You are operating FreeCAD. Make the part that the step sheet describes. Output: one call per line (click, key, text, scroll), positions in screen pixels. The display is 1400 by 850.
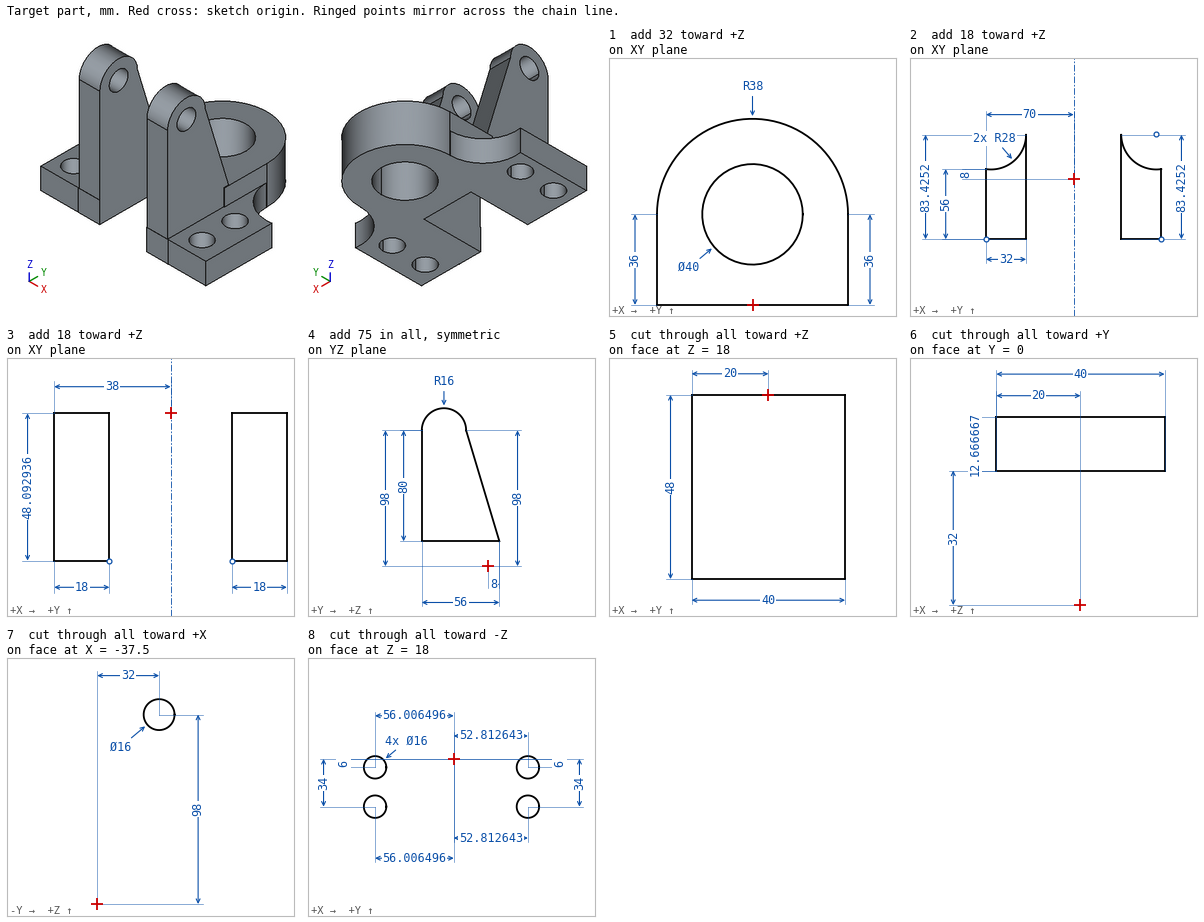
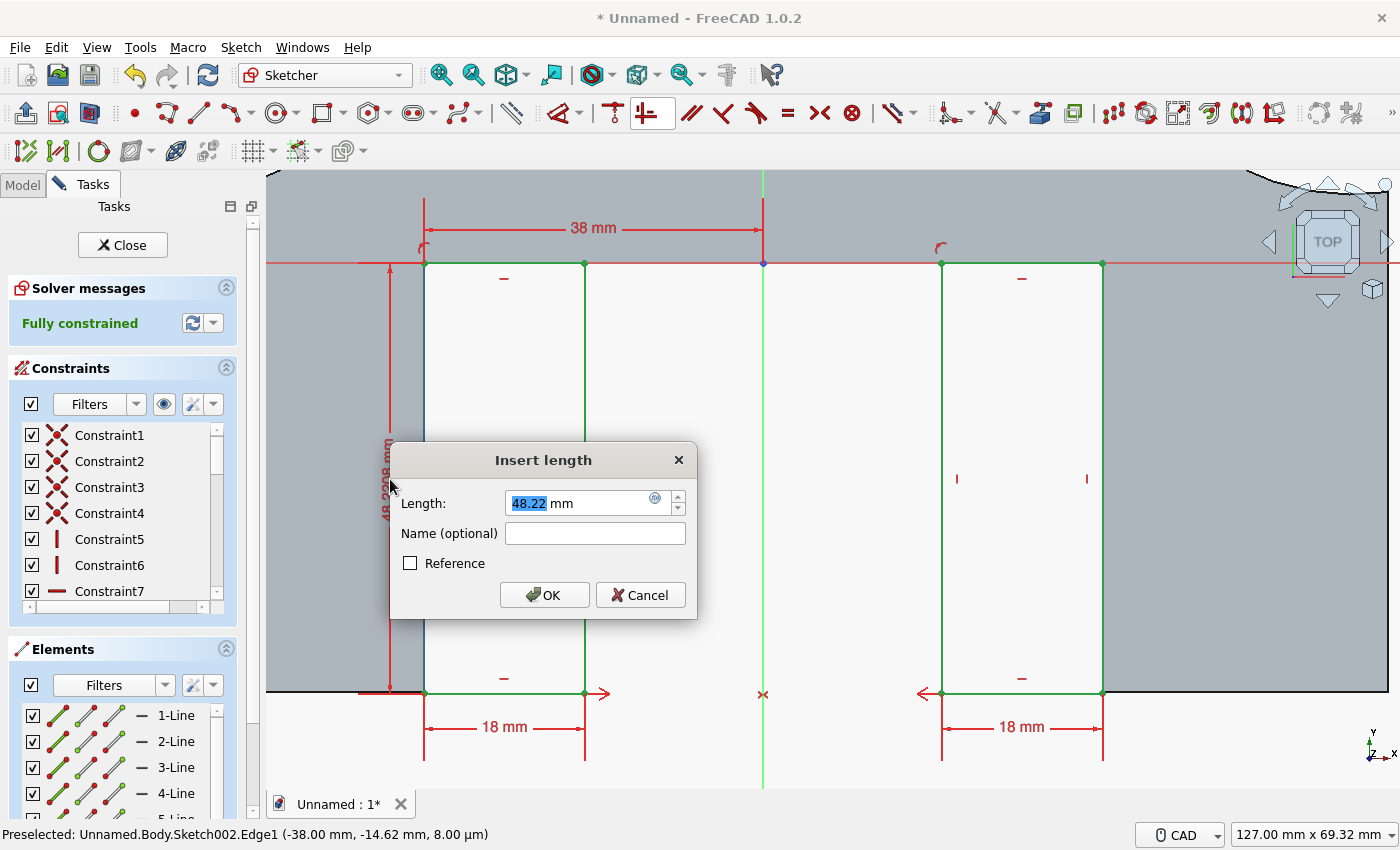
text(48.092936)
key(Return)
key(Escape)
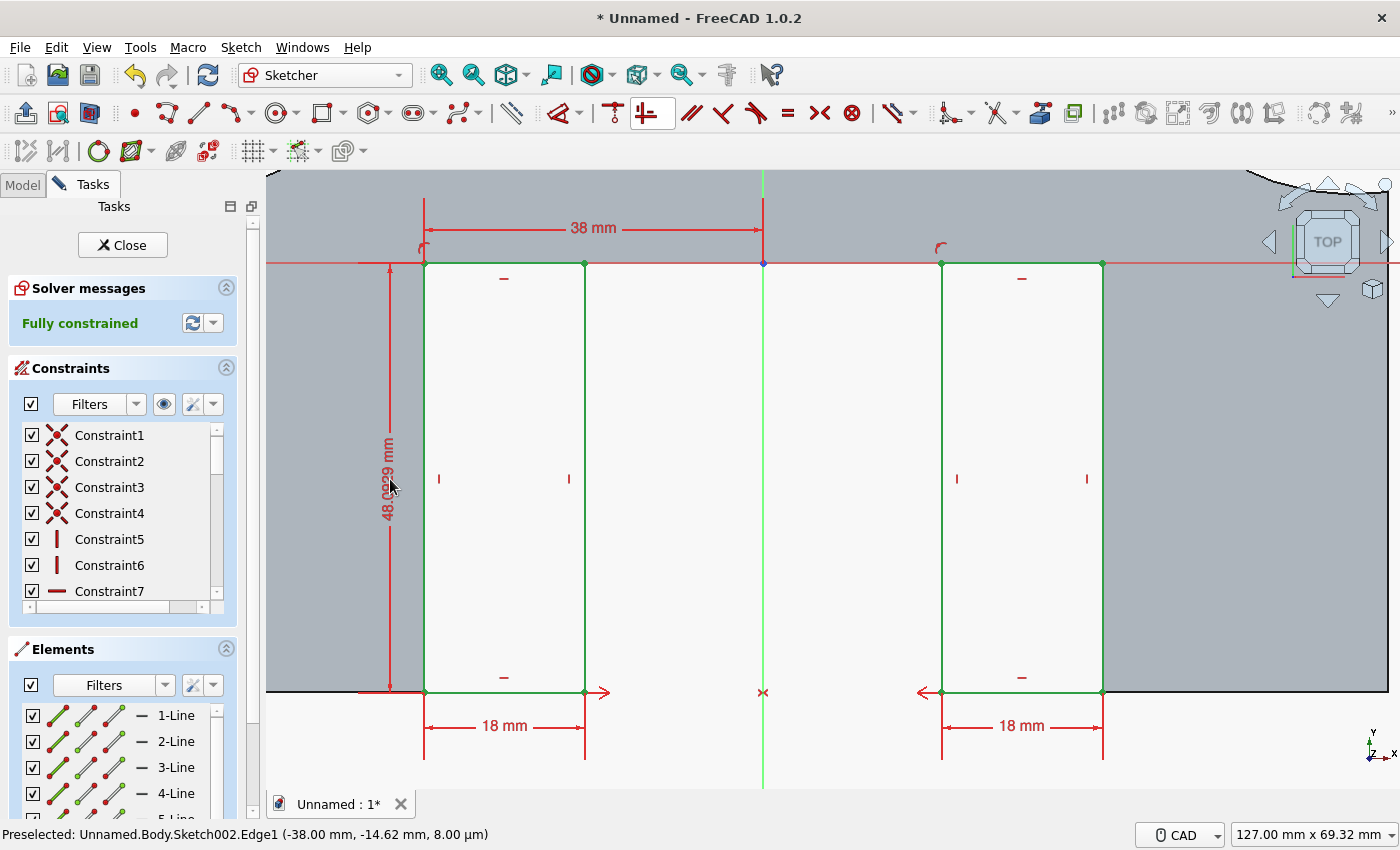
click(123, 245)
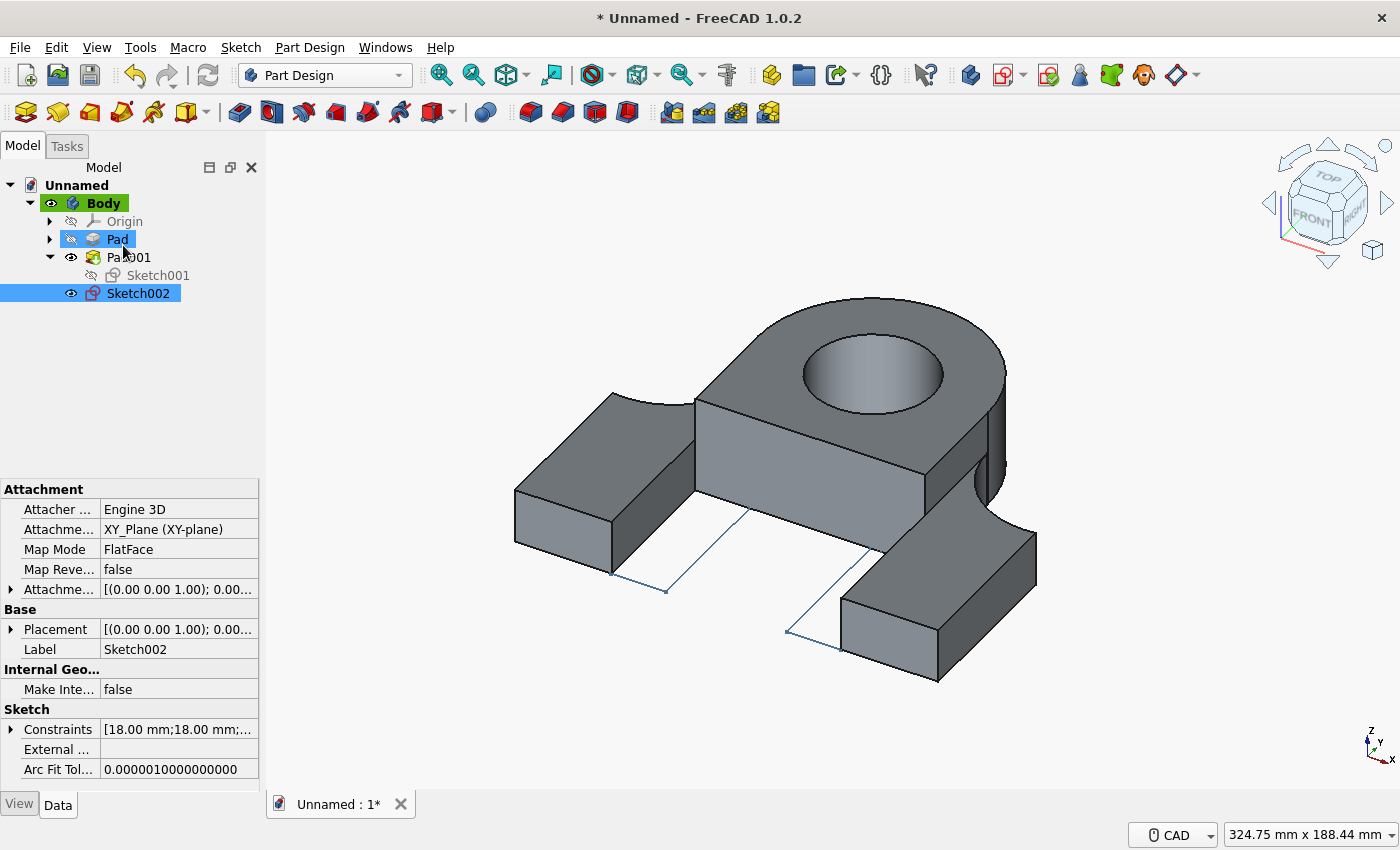
click(26, 112)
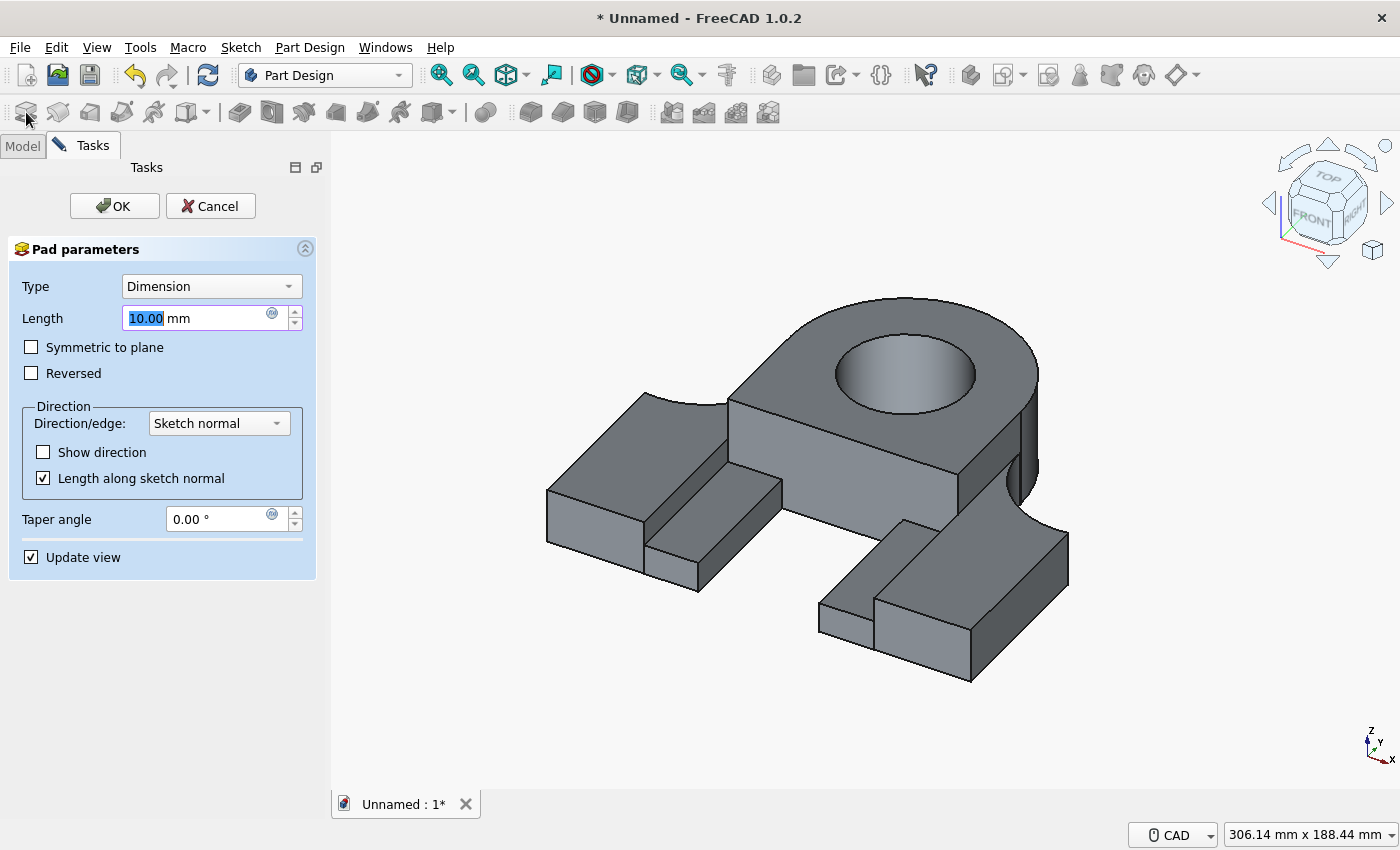
text(18)
key(Tab)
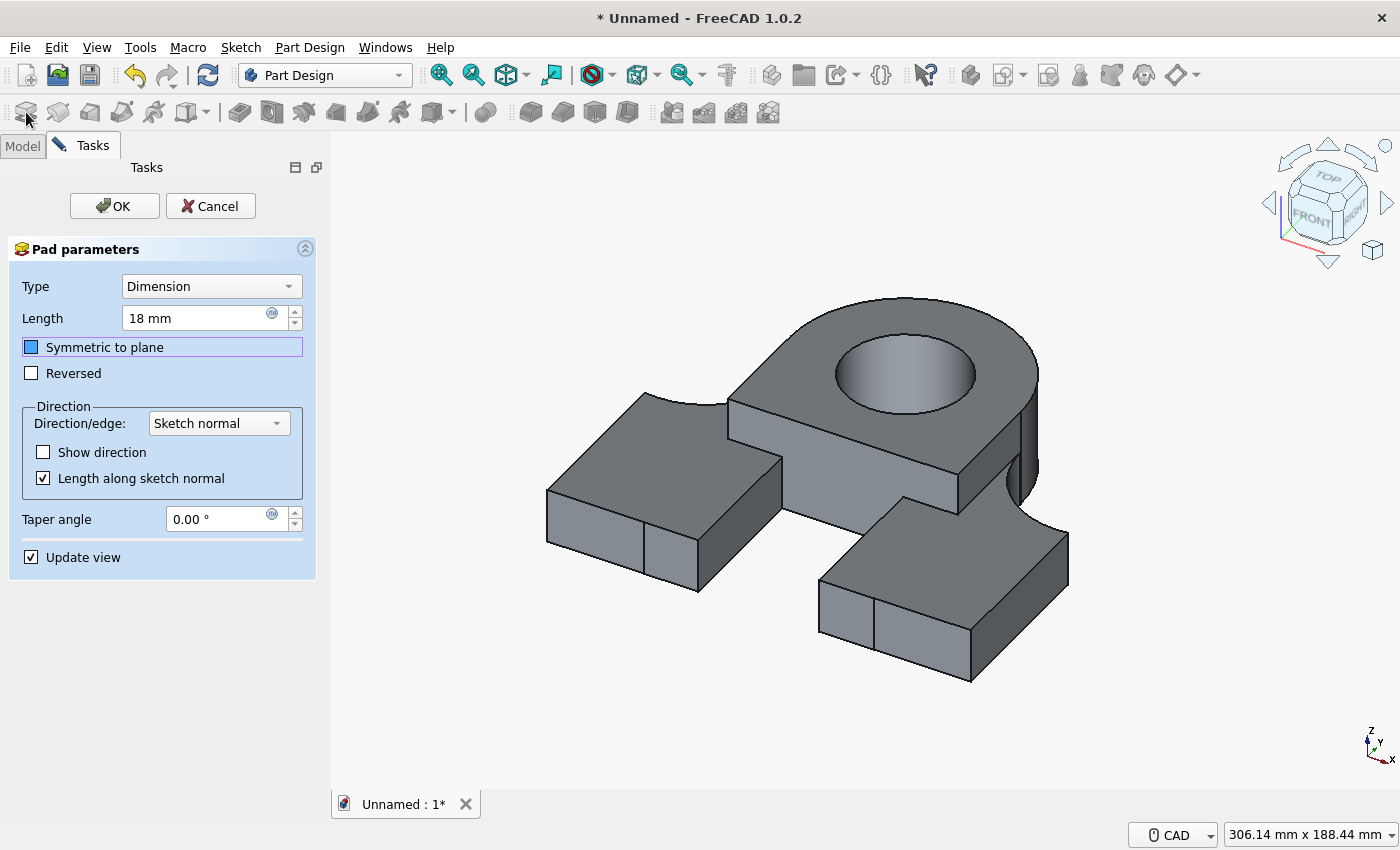
click(115, 206)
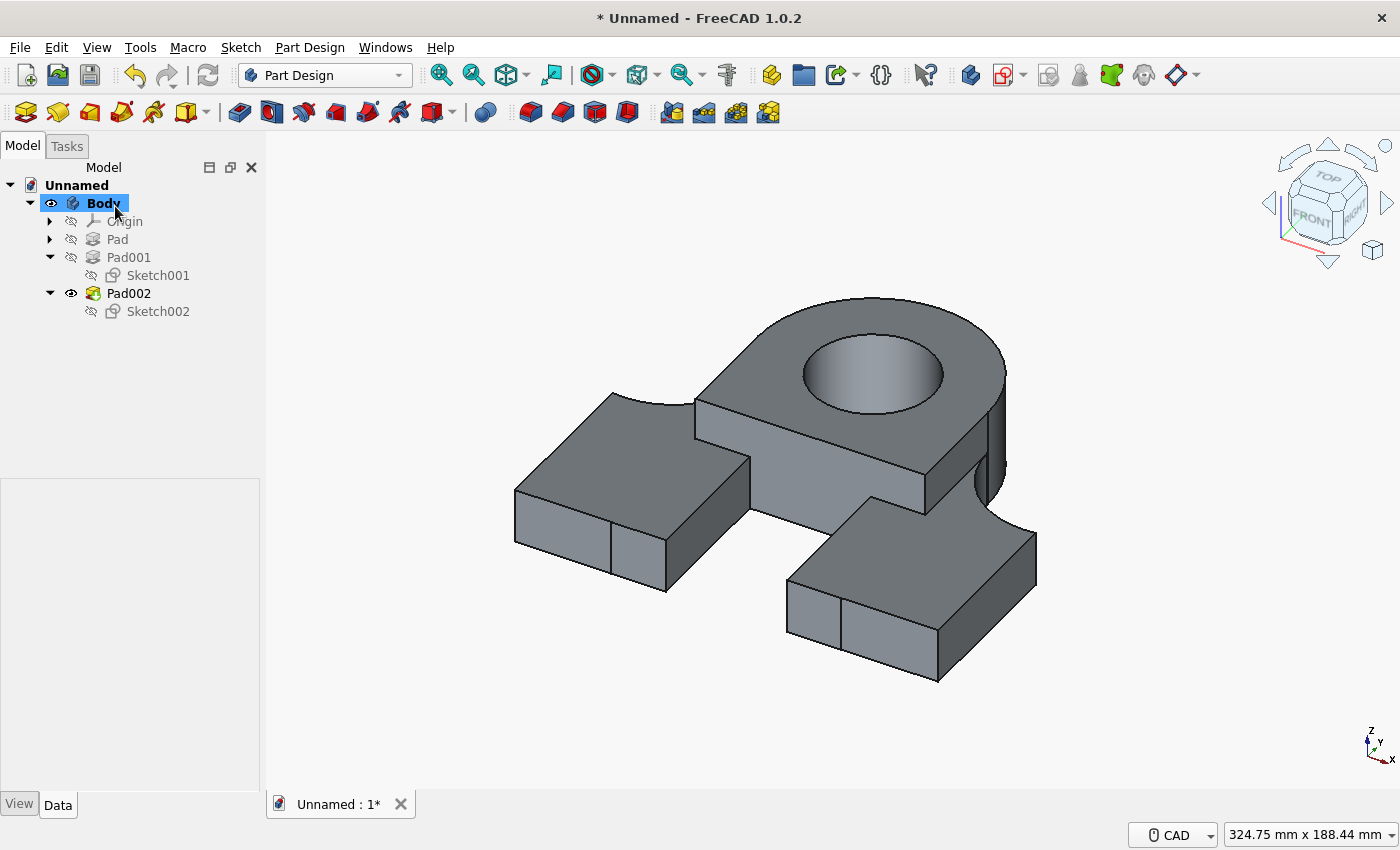
click(1004, 76)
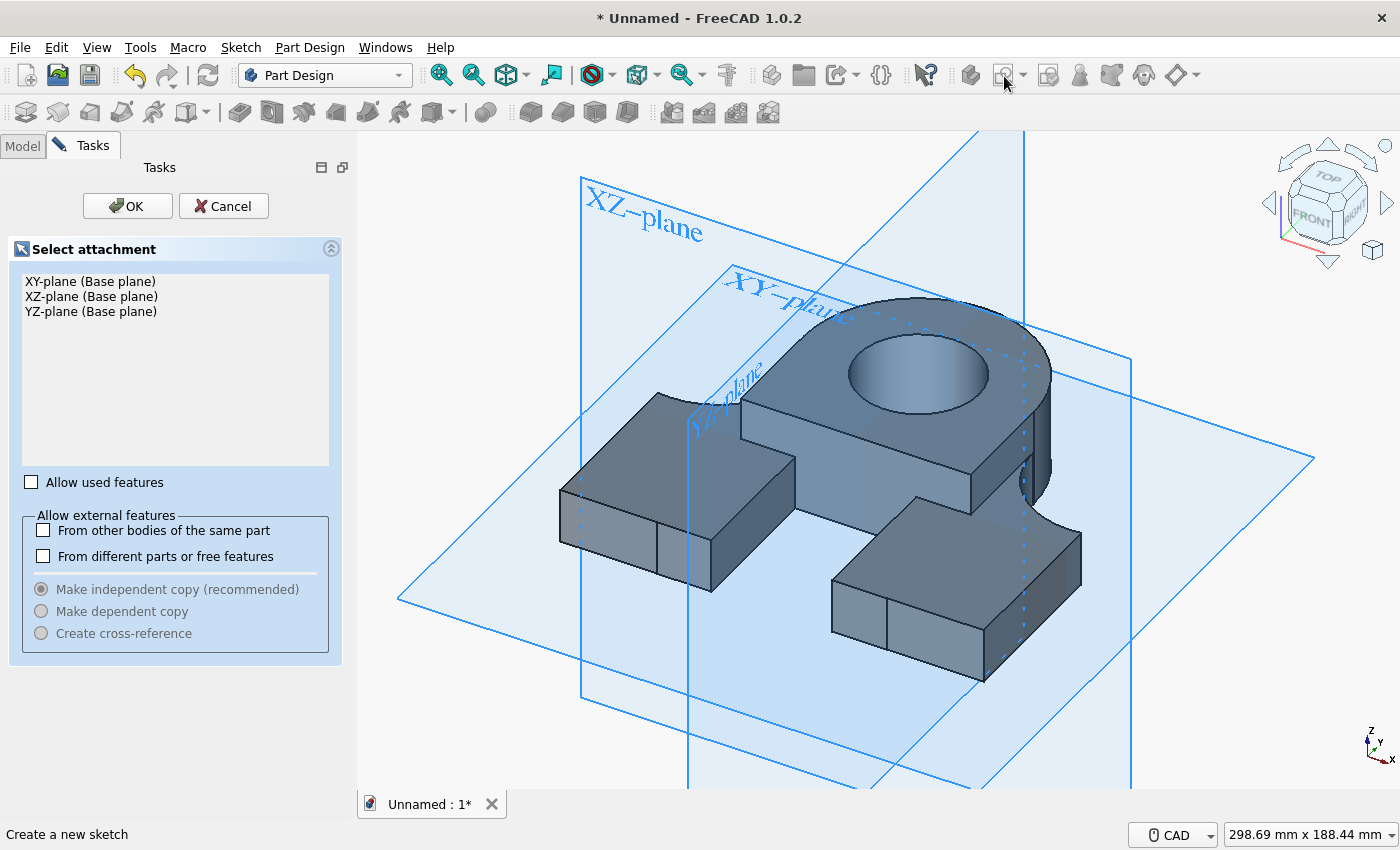
click(82, 312)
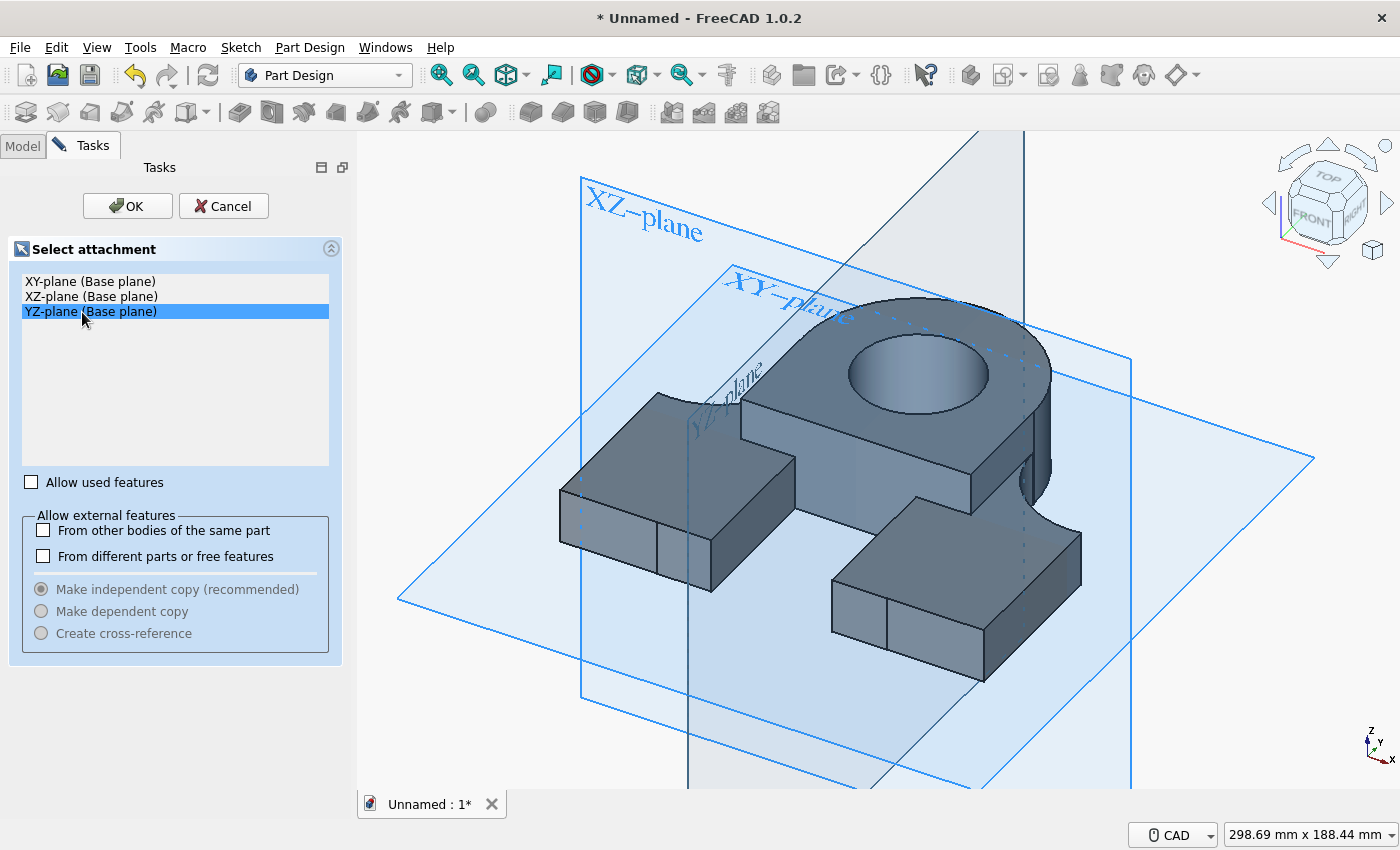
click(128, 206)